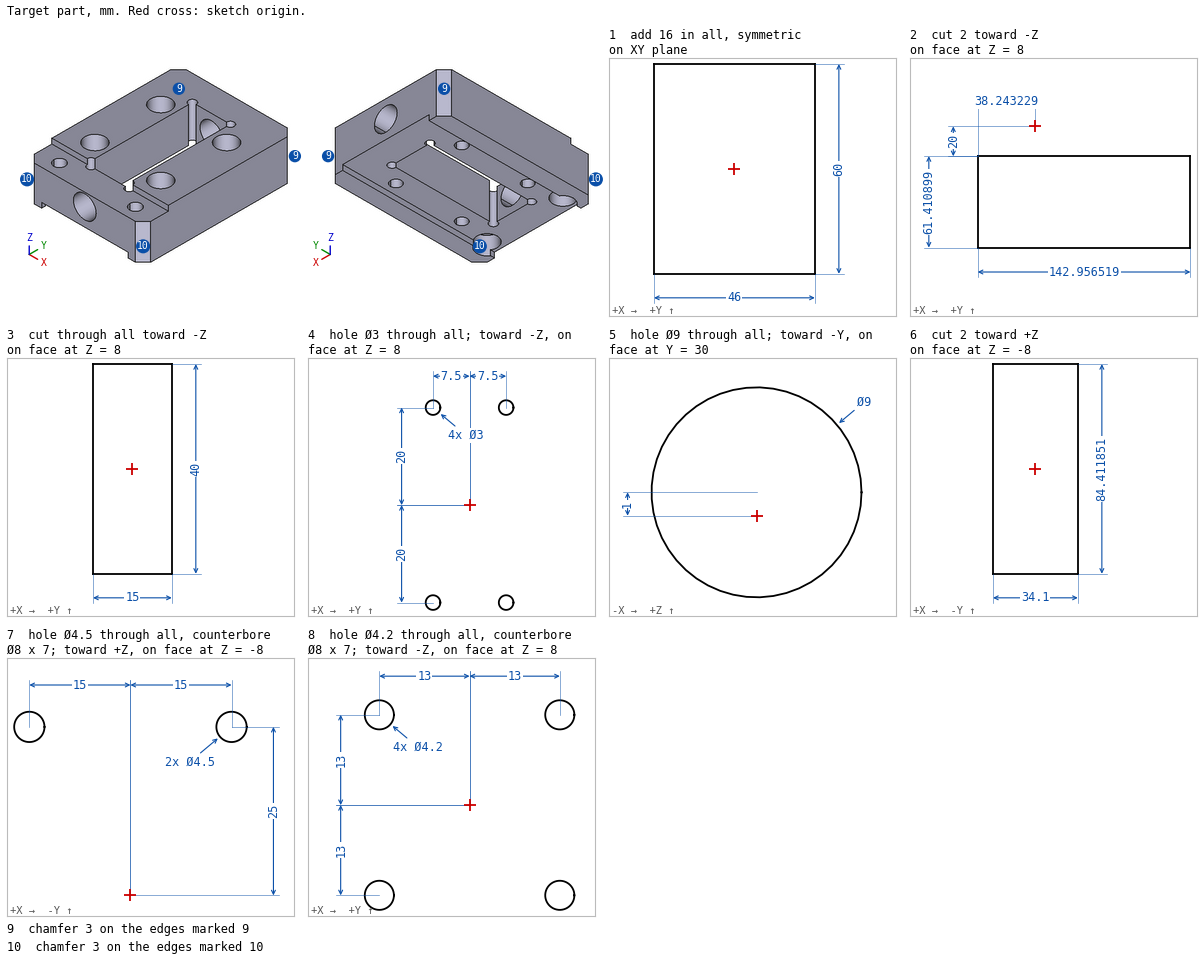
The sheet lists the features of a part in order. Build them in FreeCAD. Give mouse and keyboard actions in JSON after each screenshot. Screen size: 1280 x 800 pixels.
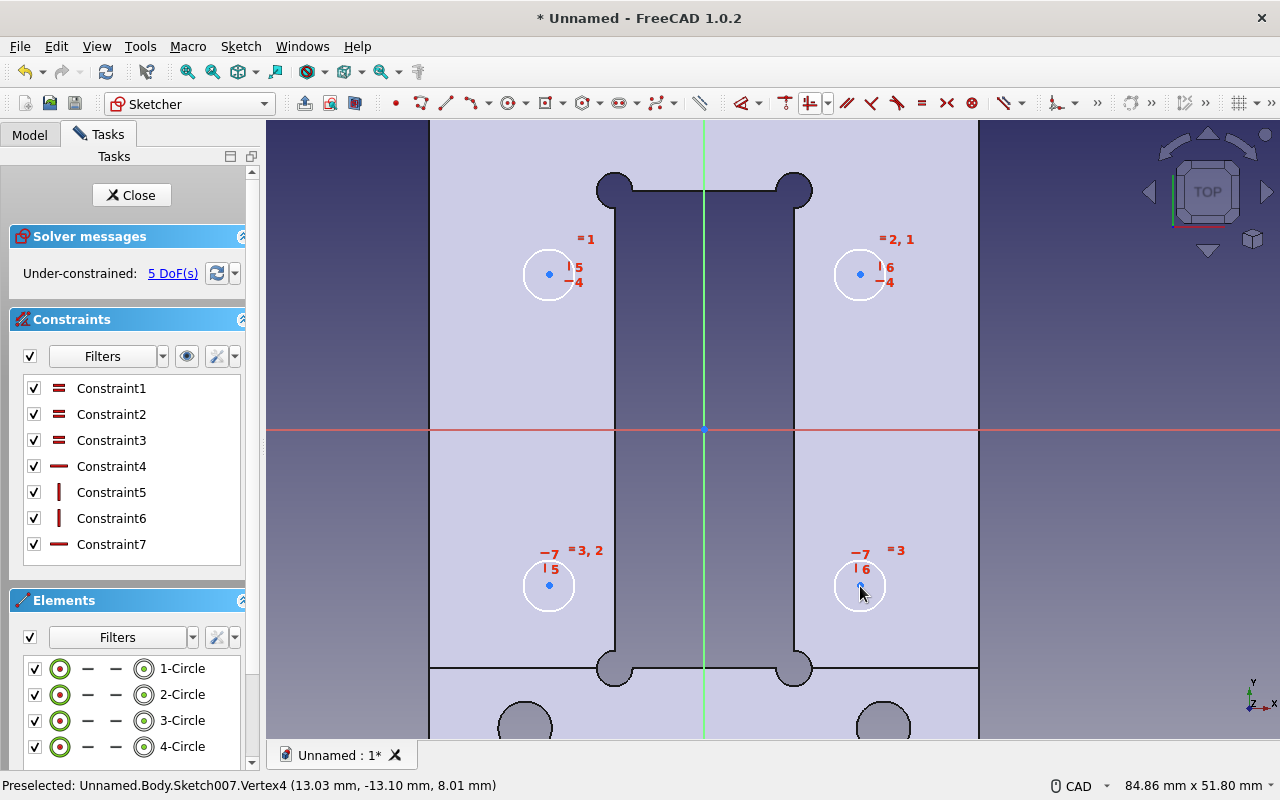
{"action": "left_click", "coordinate": [740, 104]}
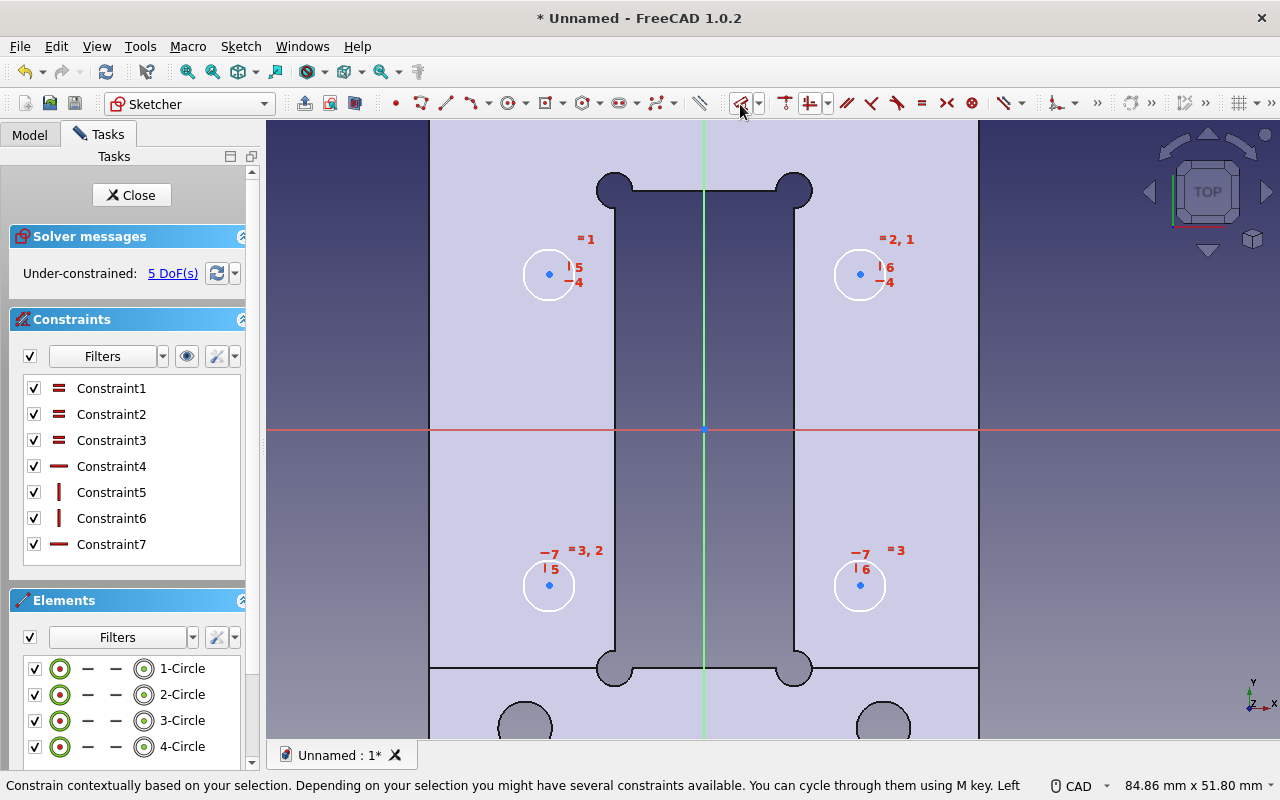
{"action": "left_click", "coordinate": [567, 257]}
{"action": "left_click", "coordinate": [590, 234]}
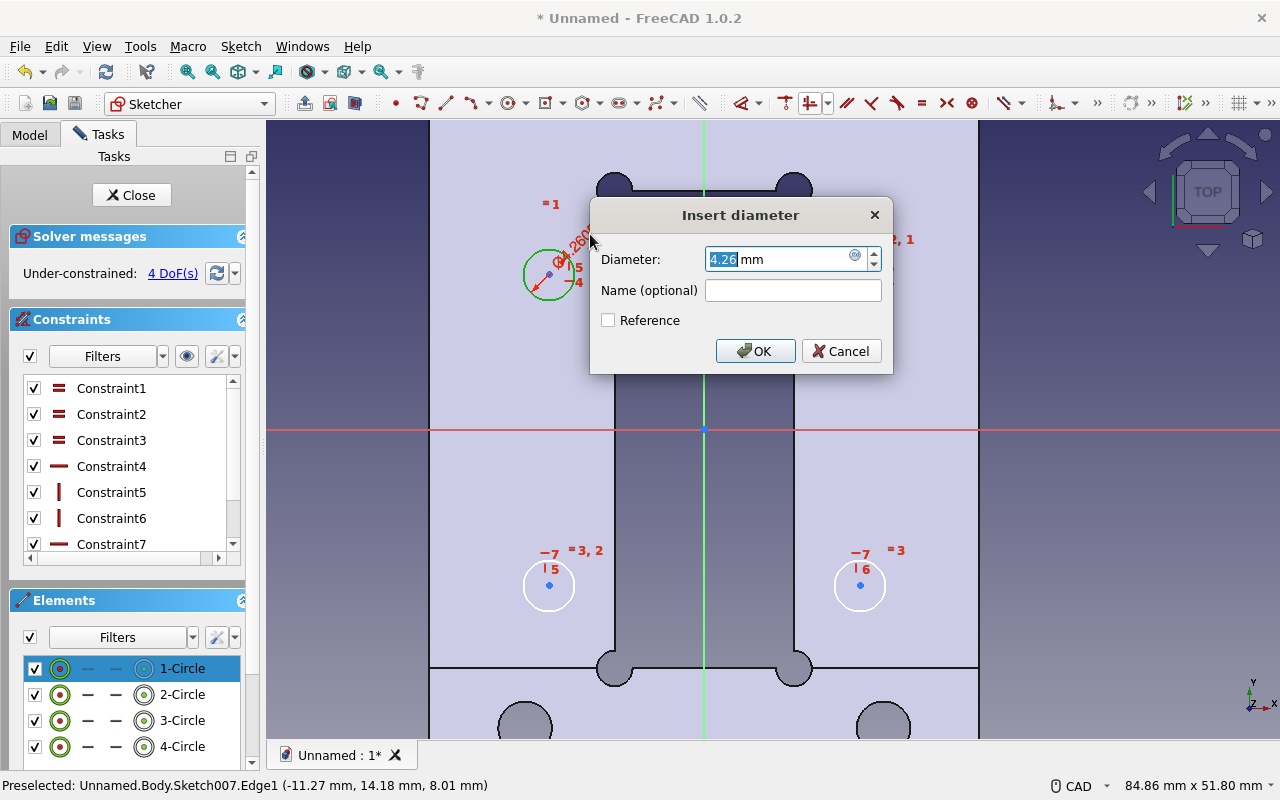
{"action": "type", "text": "4.2"}
{"action": "key", "text": "Return"}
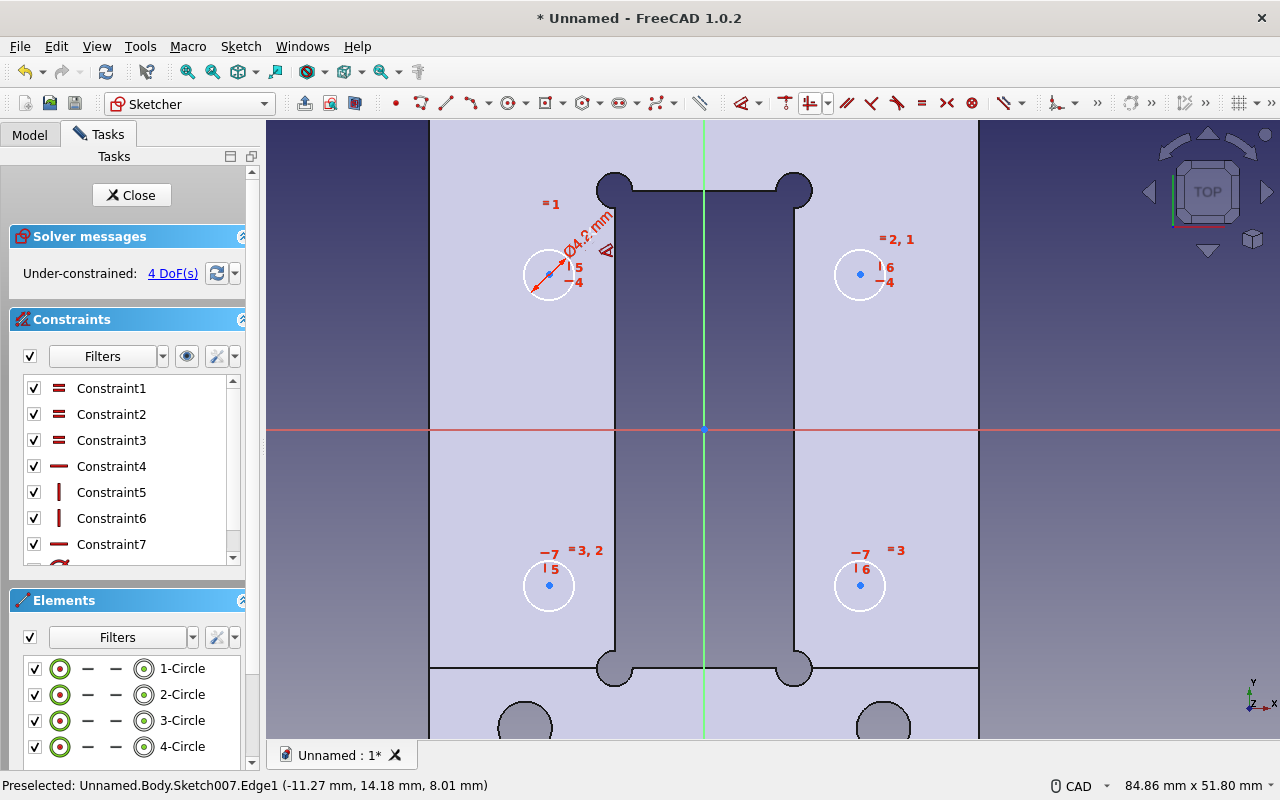
{"action": "left_click", "coordinate": [549, 275]}
{"action": "left_click", "coordinate": [662, 241]}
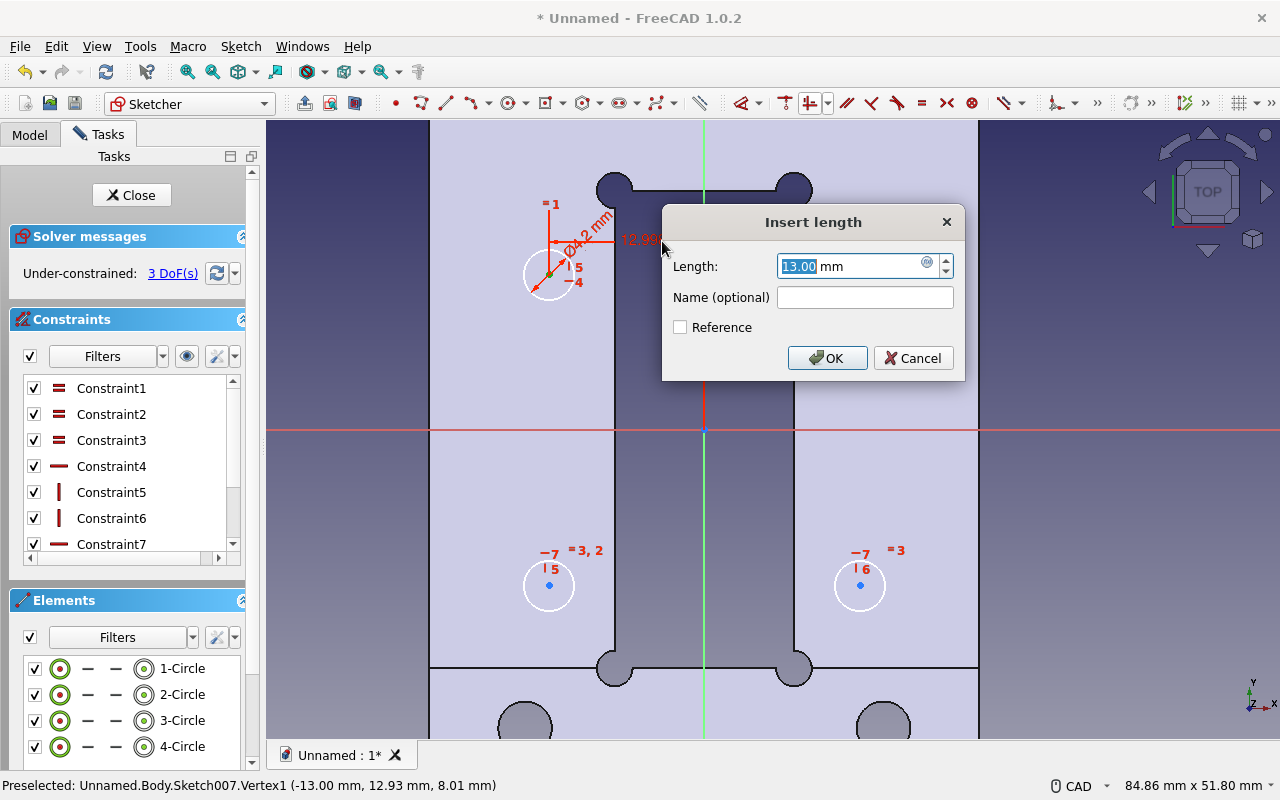
{"action": "type", "text": "13"}
{"action": "key", "text": "Return"}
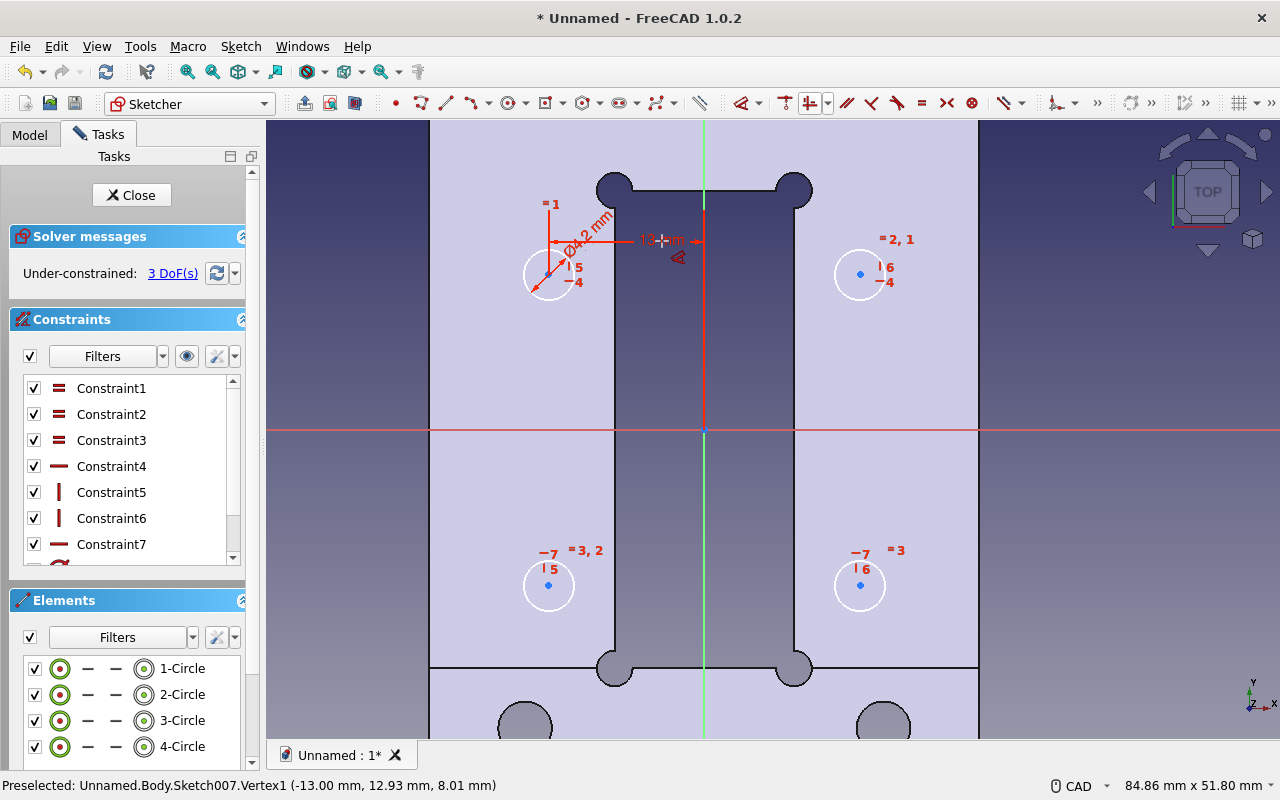
{"action": "left_click", "coordinate": [549, 275]}
{"action": "left_click", "coordinate": [515, 352]}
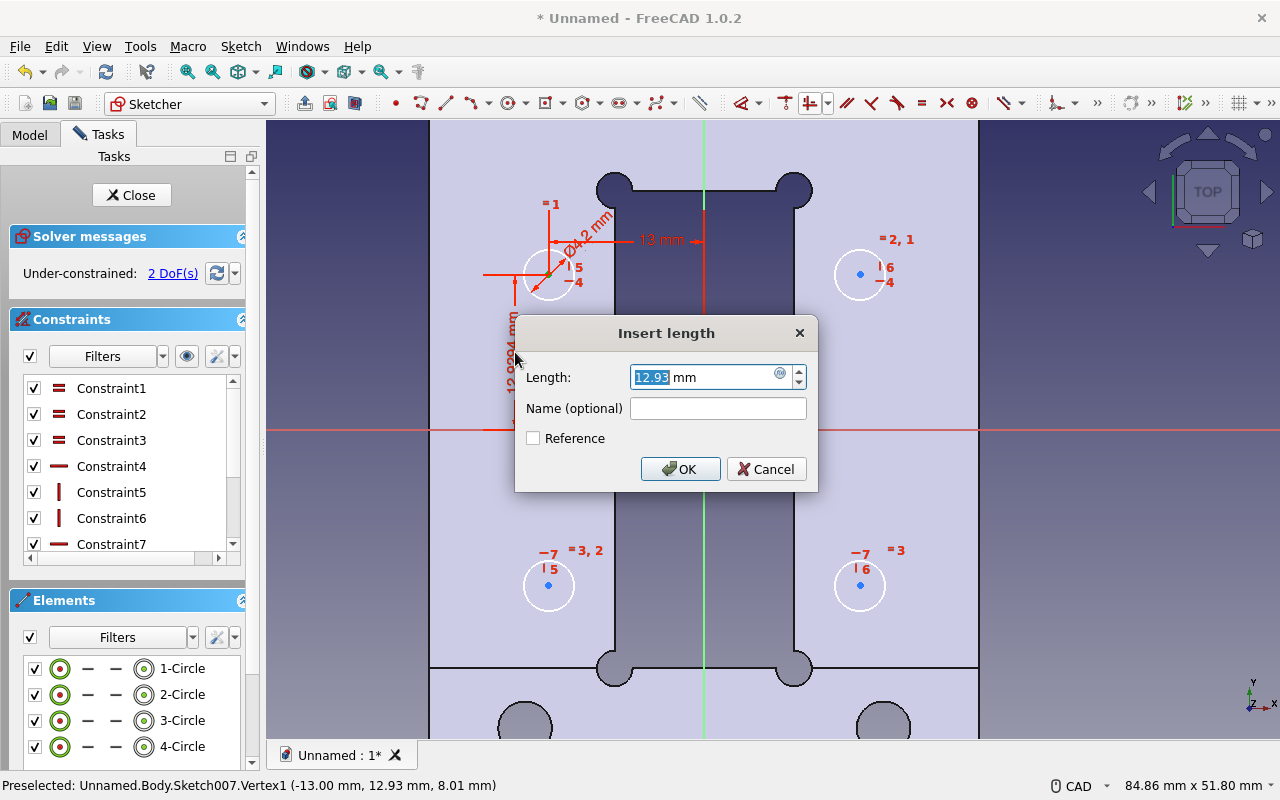
{"action": "type", "text": "13"}
{"action": "key", "text": "Return"}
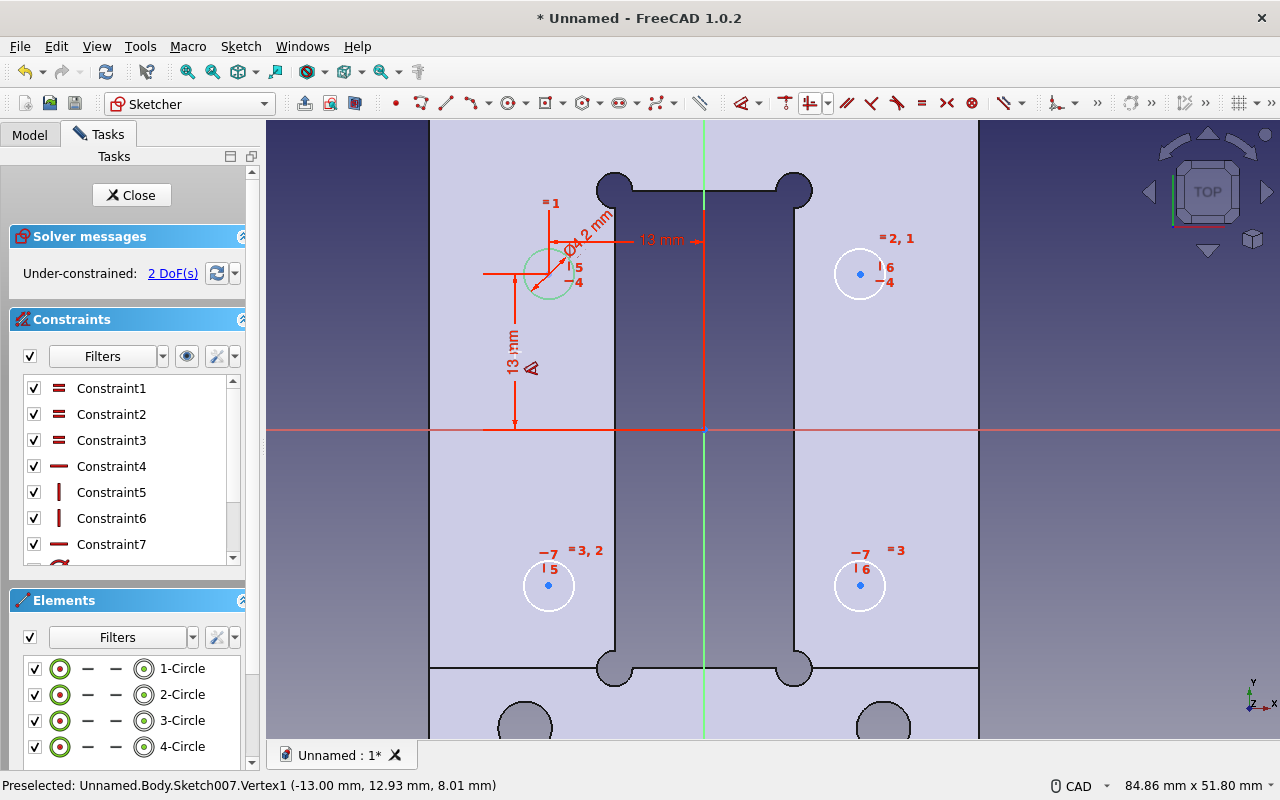
{"action": "left_click", "coordinate": [860, 274]}
{"action": "left_click", "coordinate": [782, 240]}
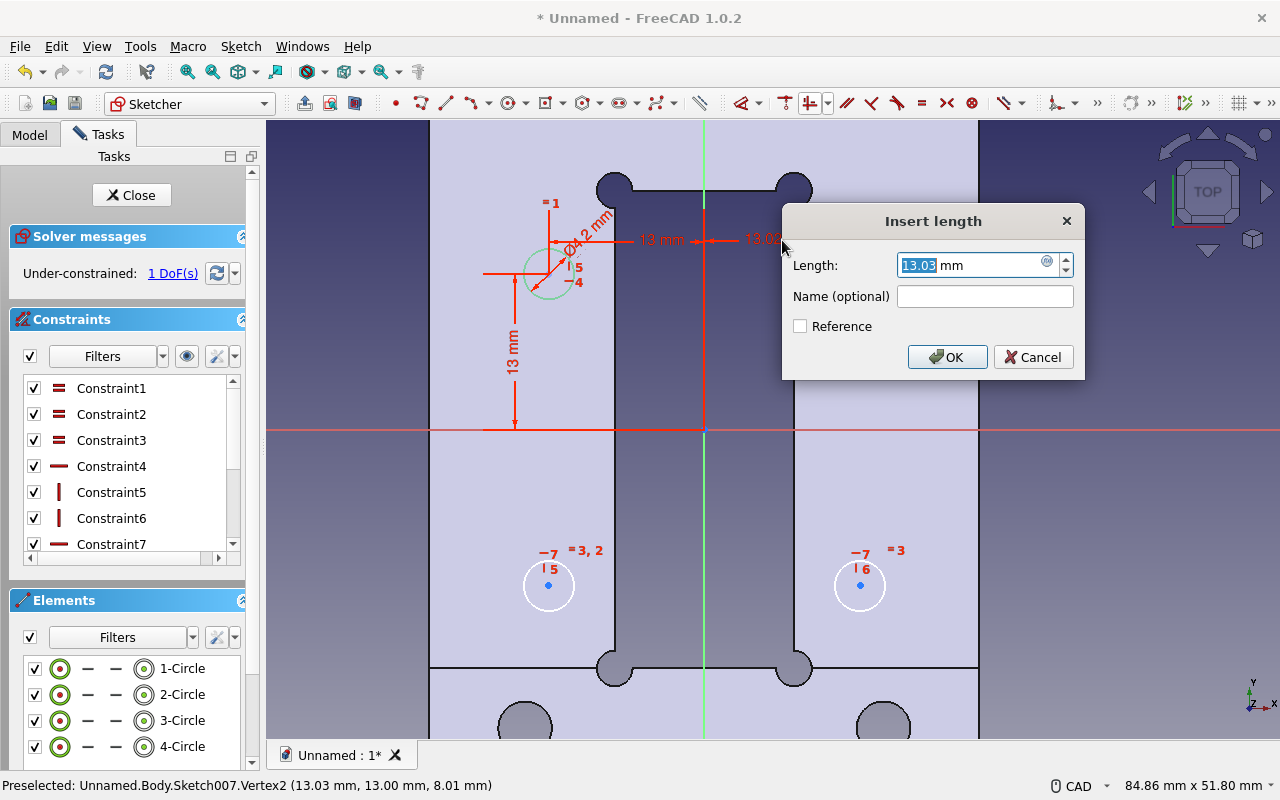
{"action": "type", "text": "13"}
{"action": "key", "text": "Return"}